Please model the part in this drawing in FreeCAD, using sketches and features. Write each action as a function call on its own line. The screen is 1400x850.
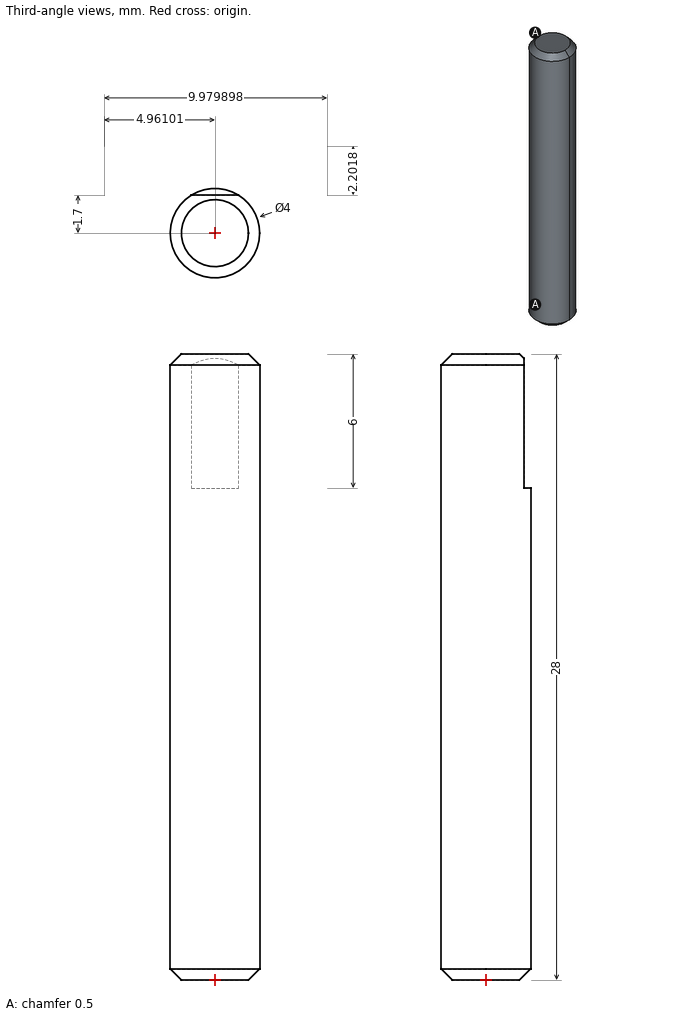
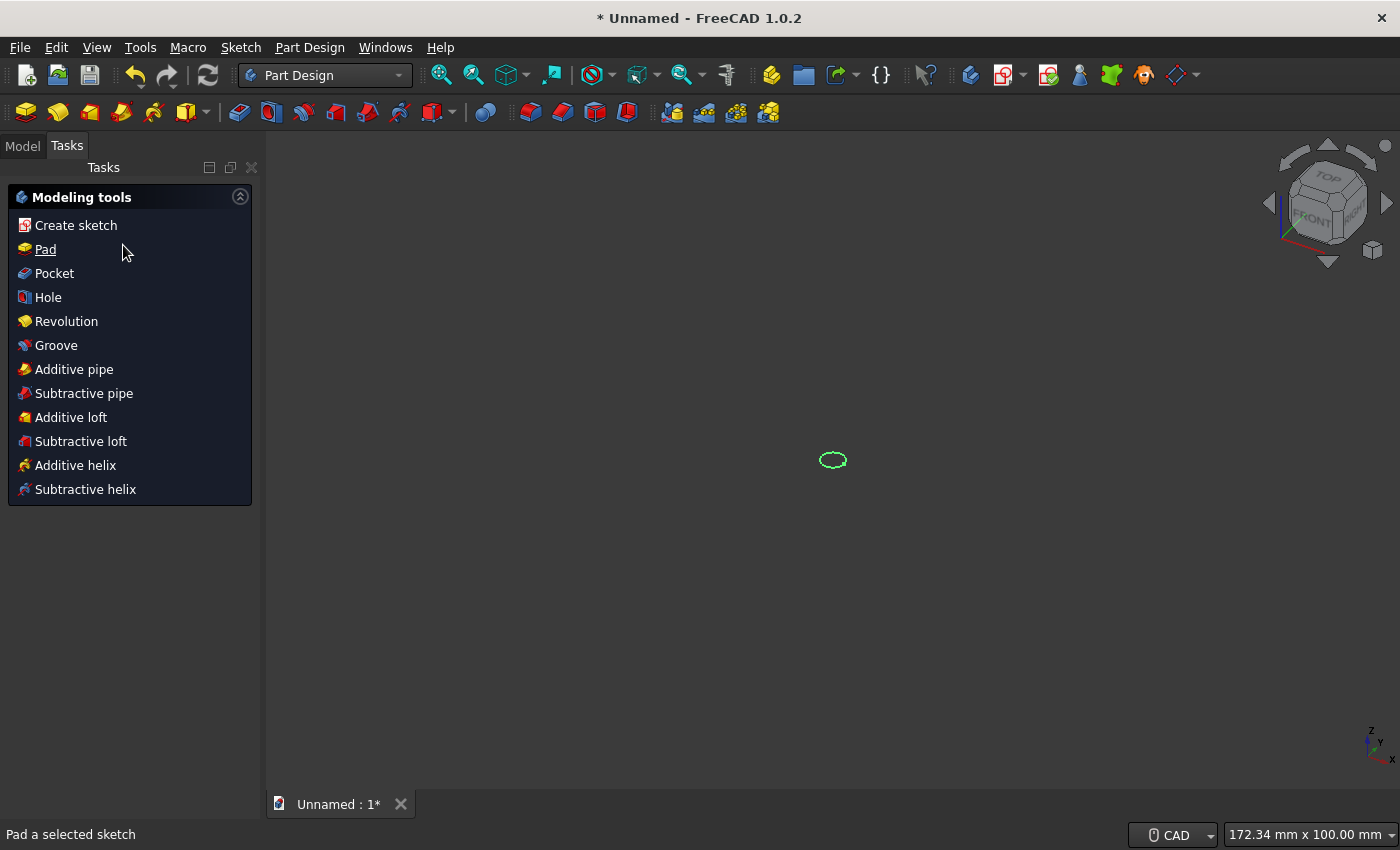
click(26, 112)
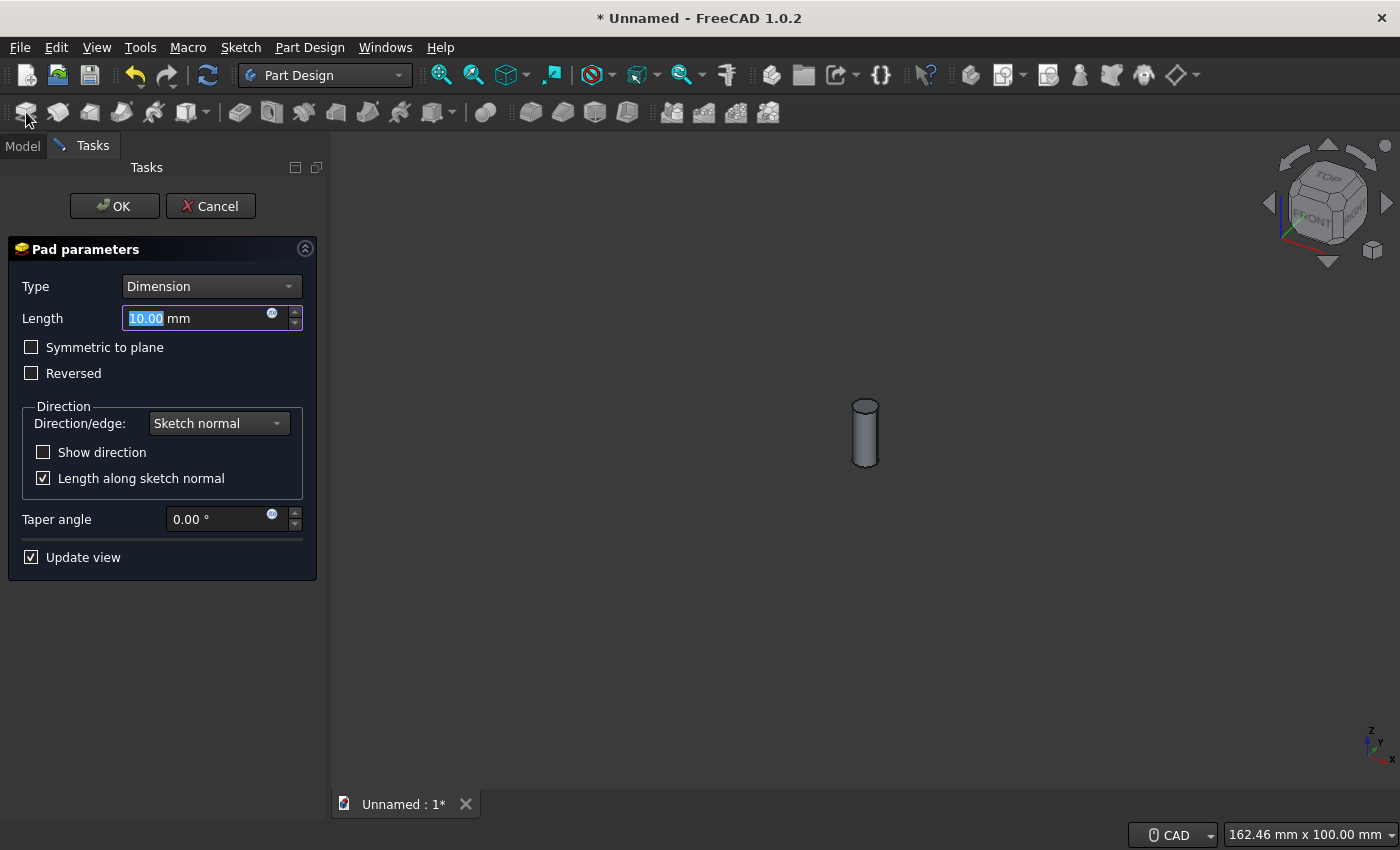
text(28)
key(Tab)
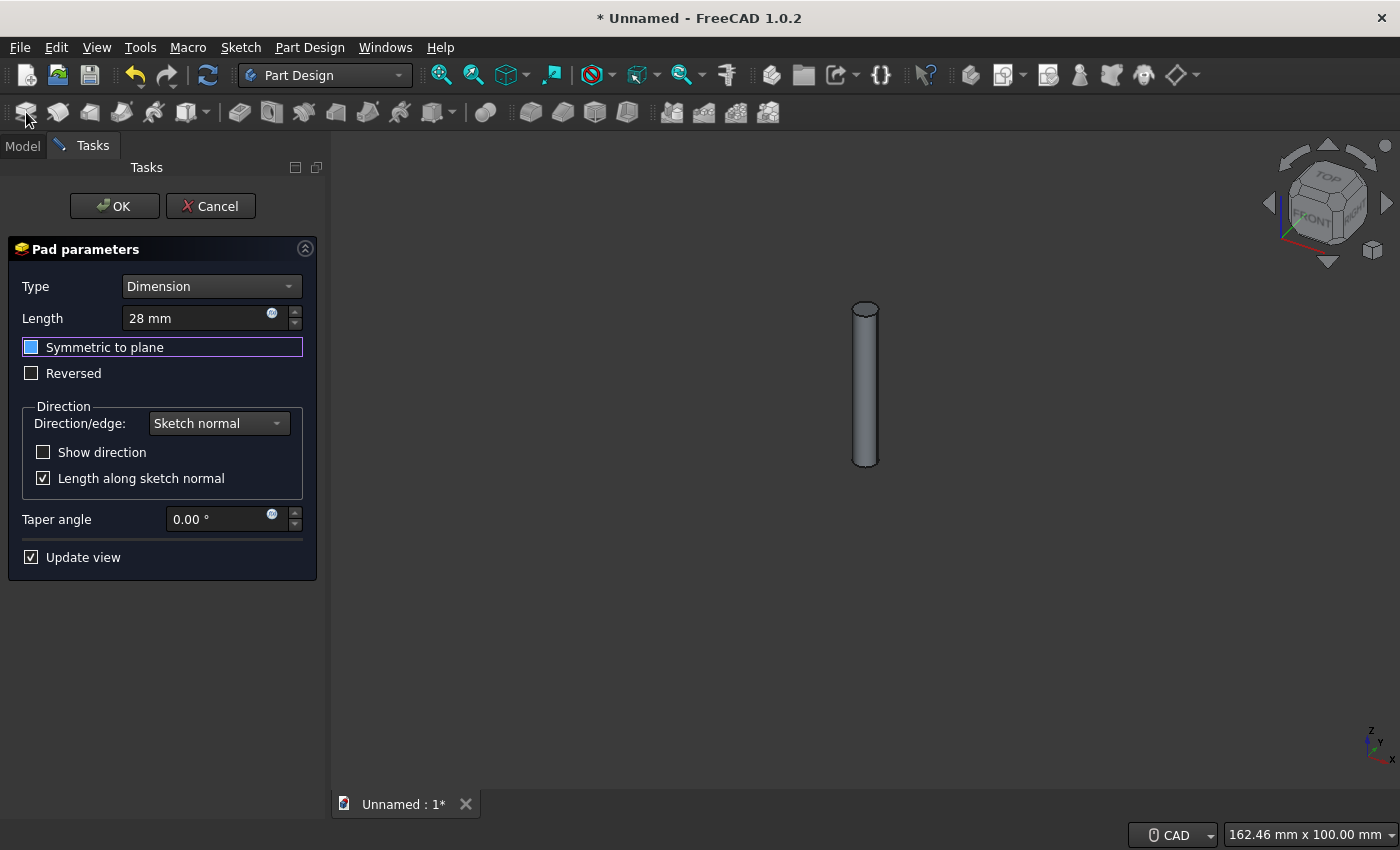
click(115, 206)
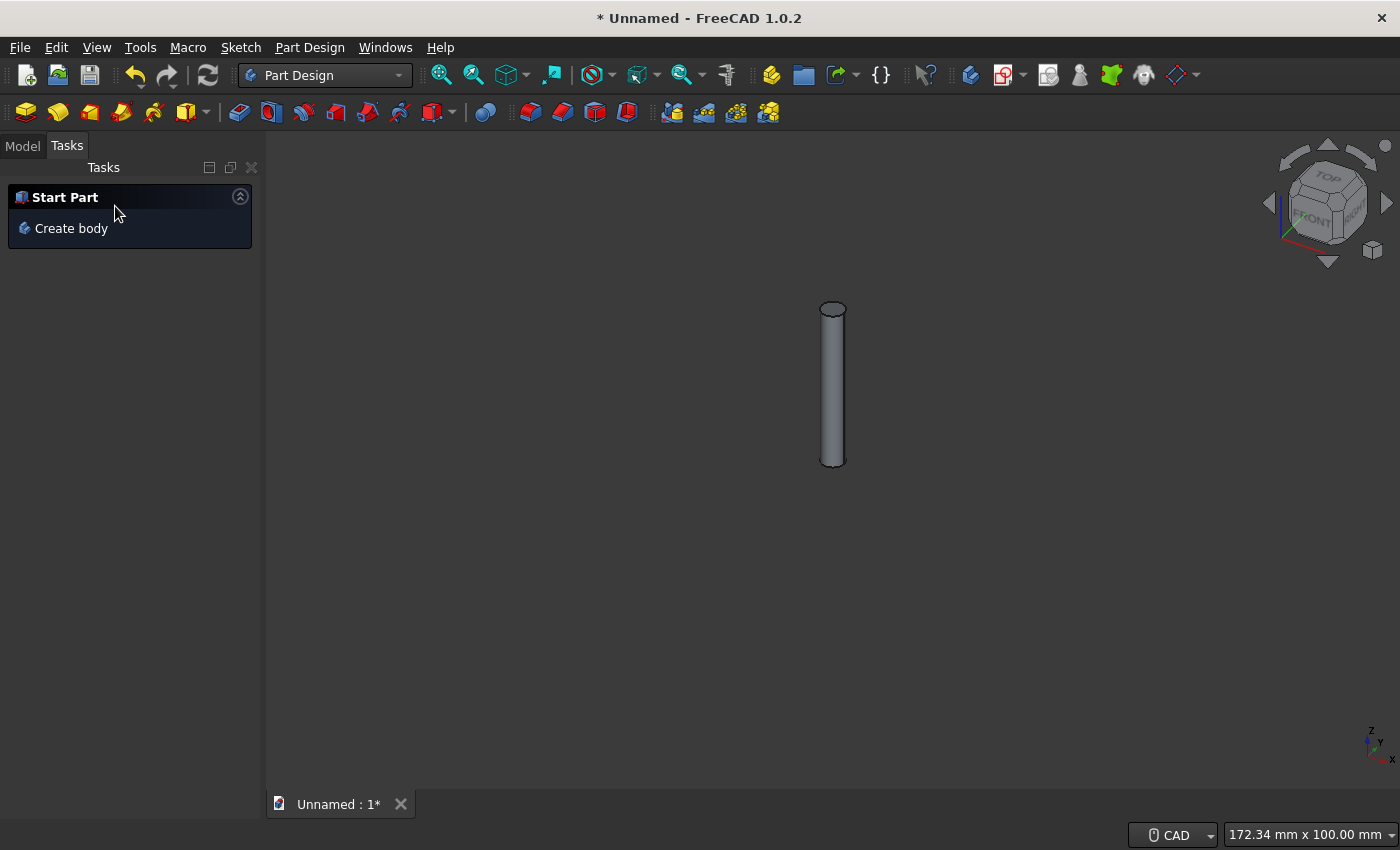
click(442, 76)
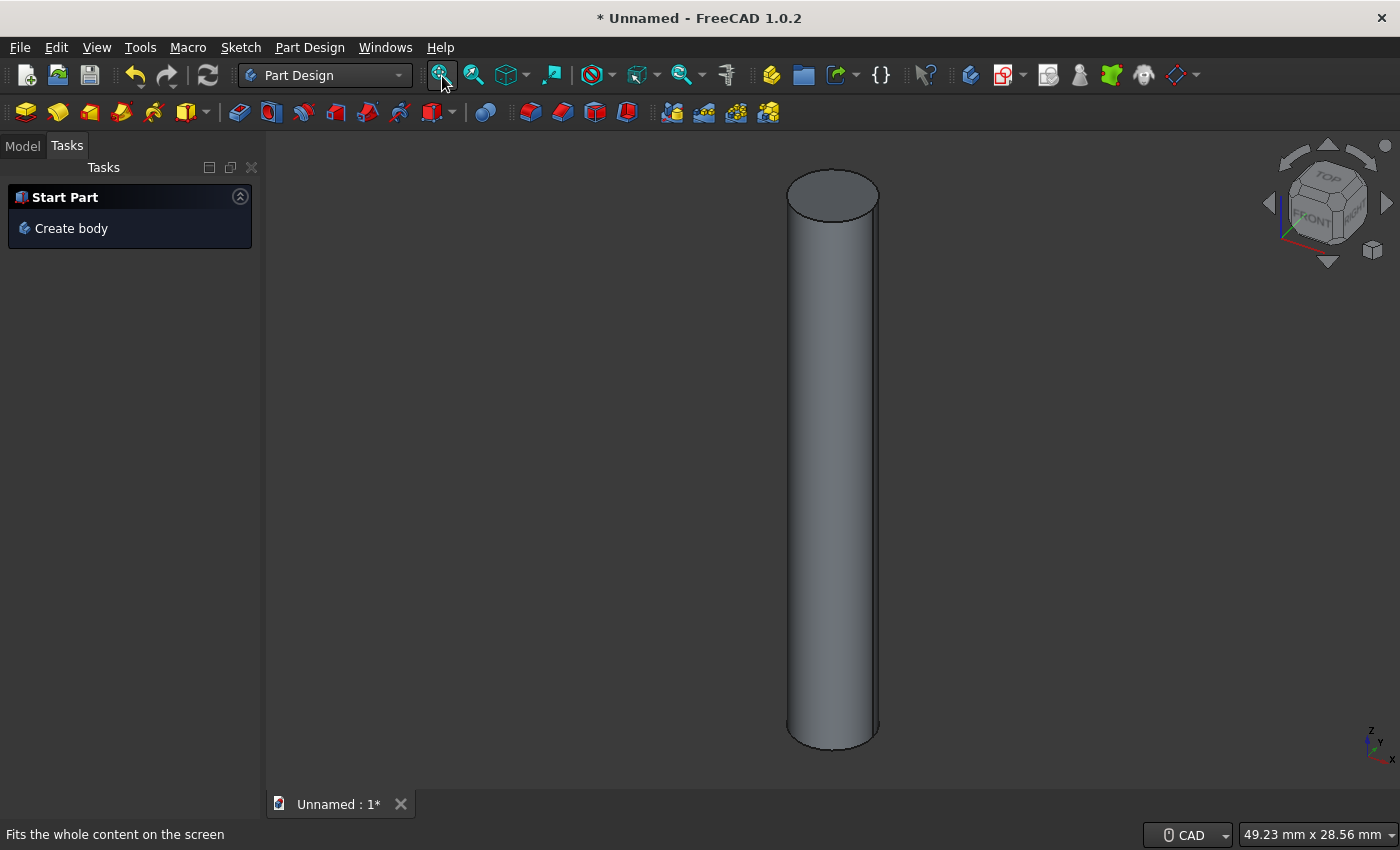
click(787, 198)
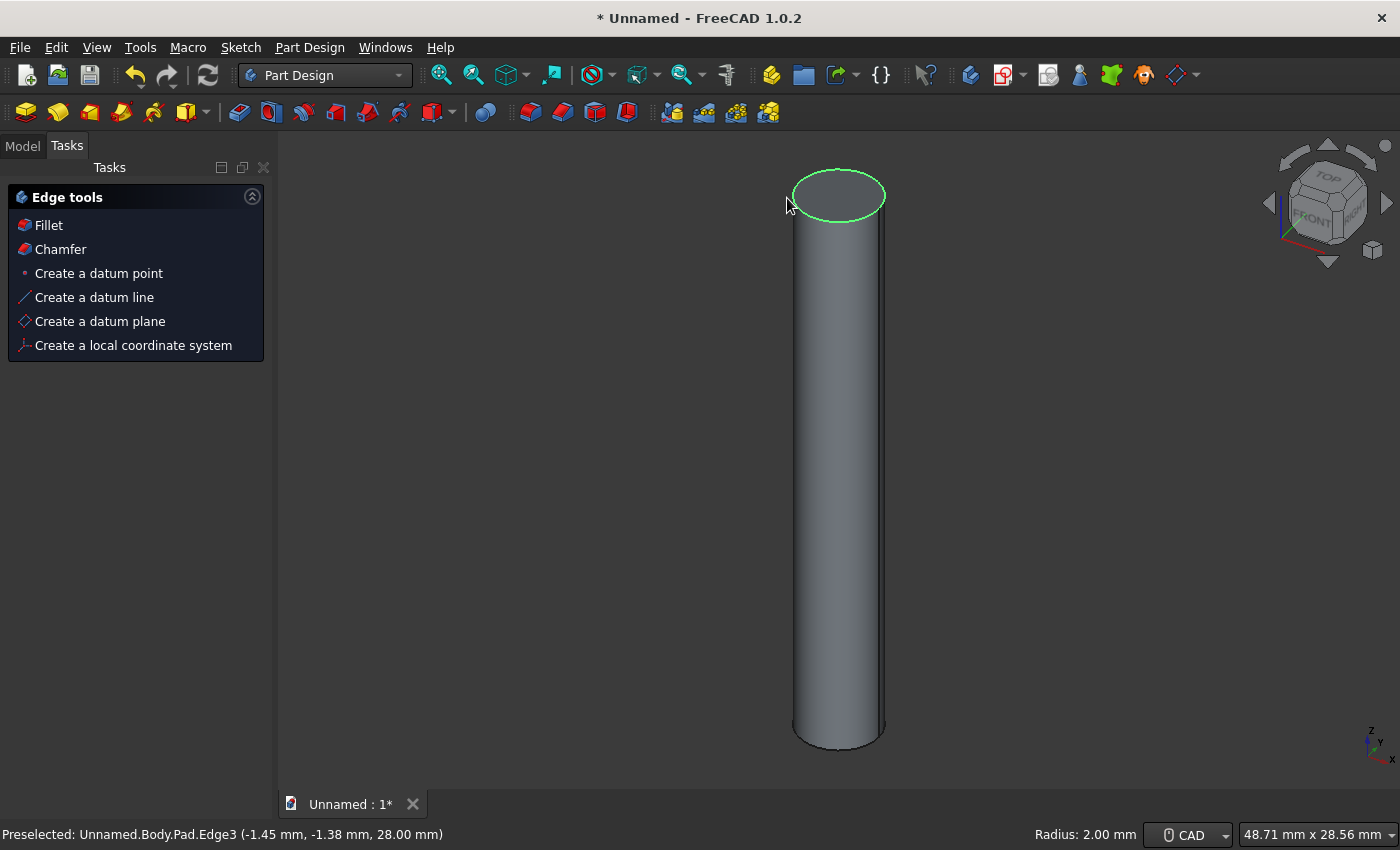
key(0)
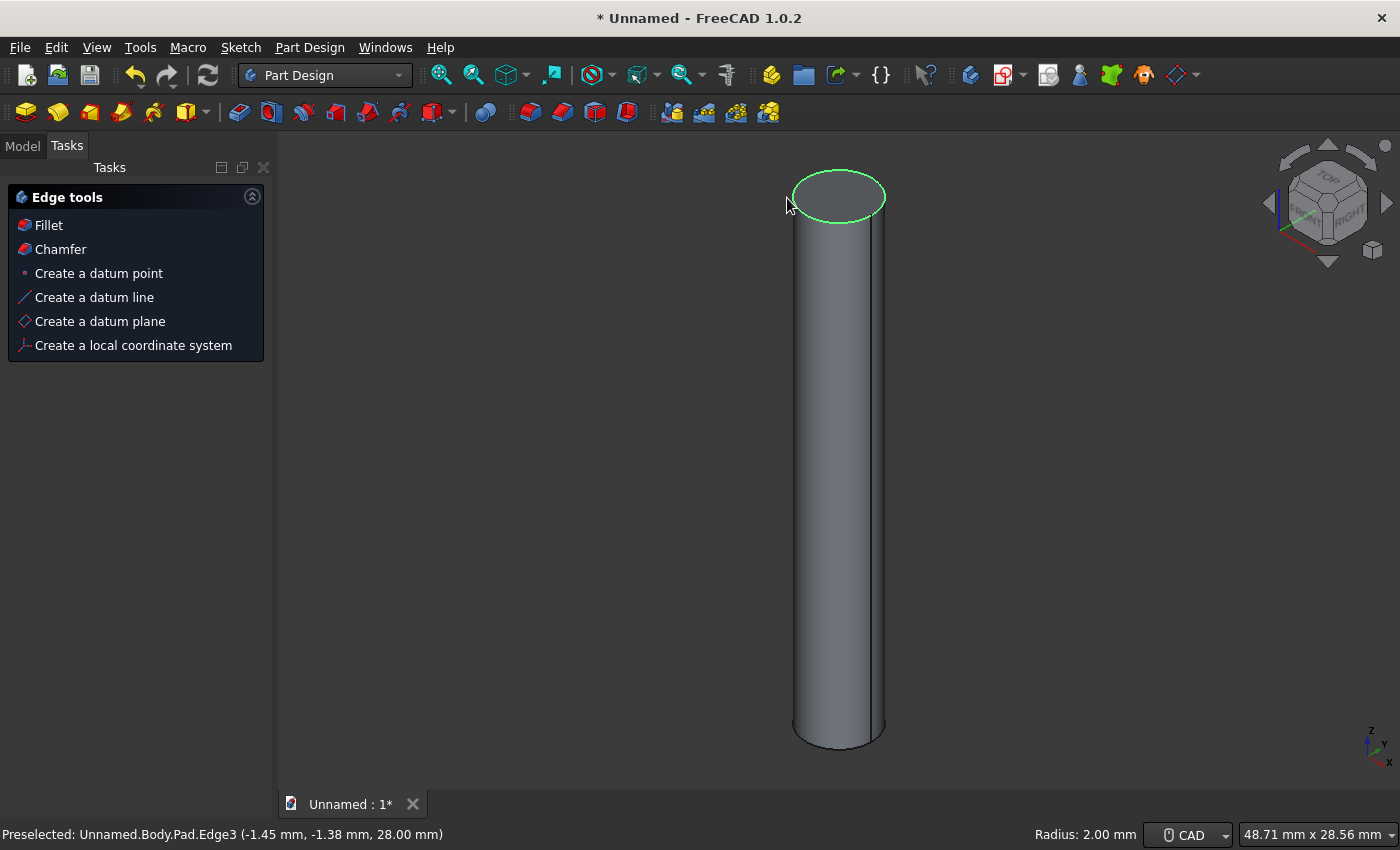
key(2)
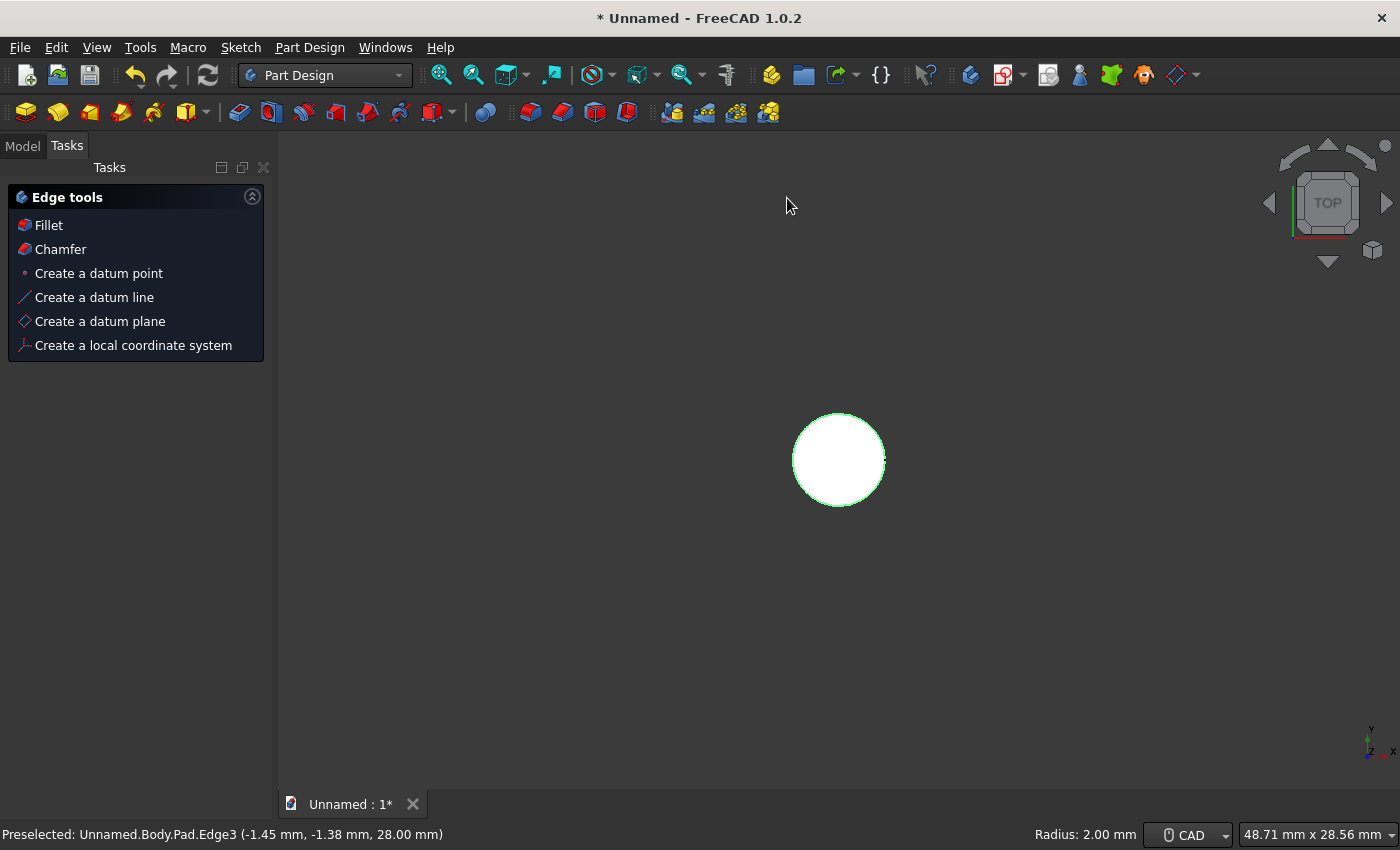
click(442, 76)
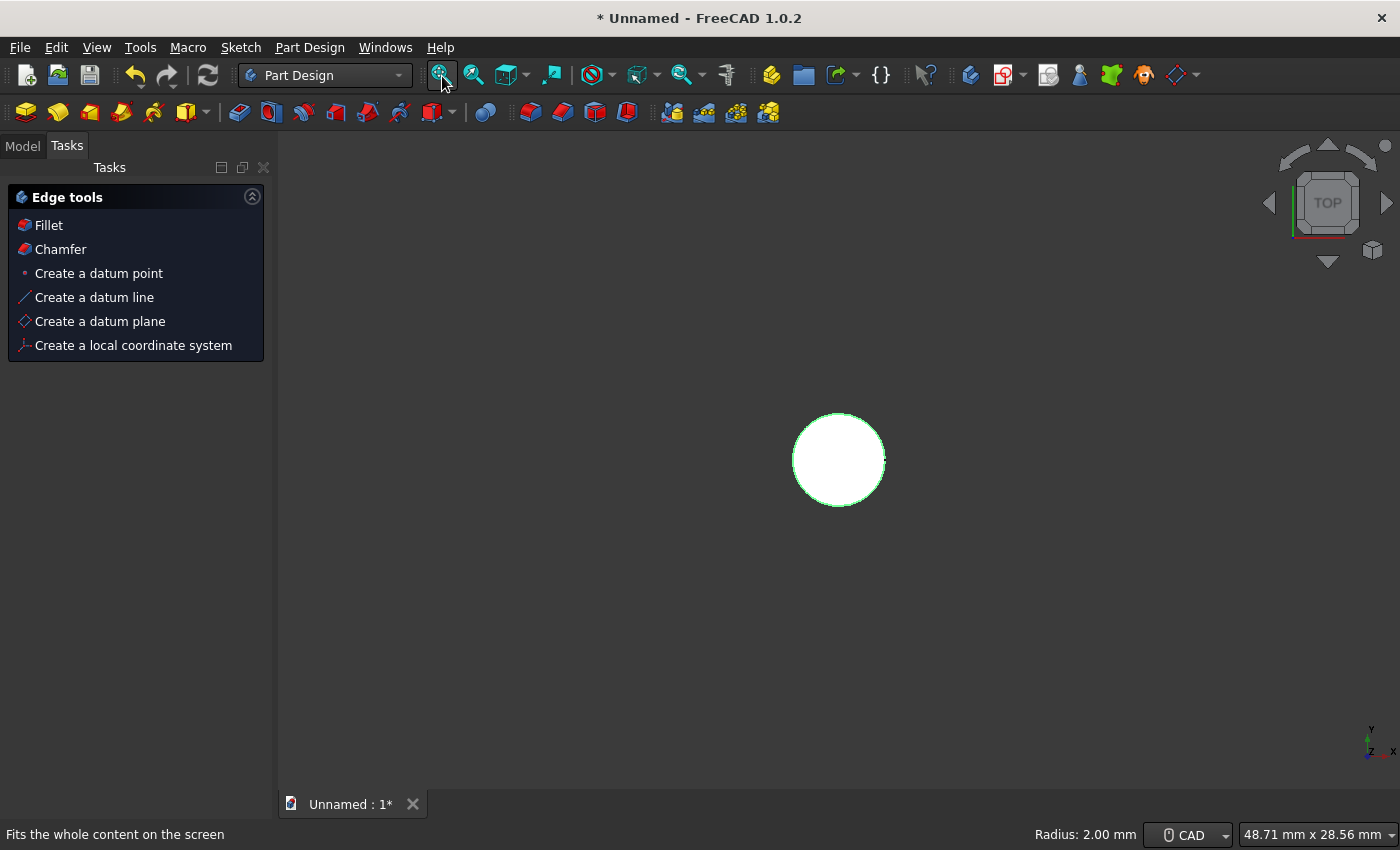
key(1)